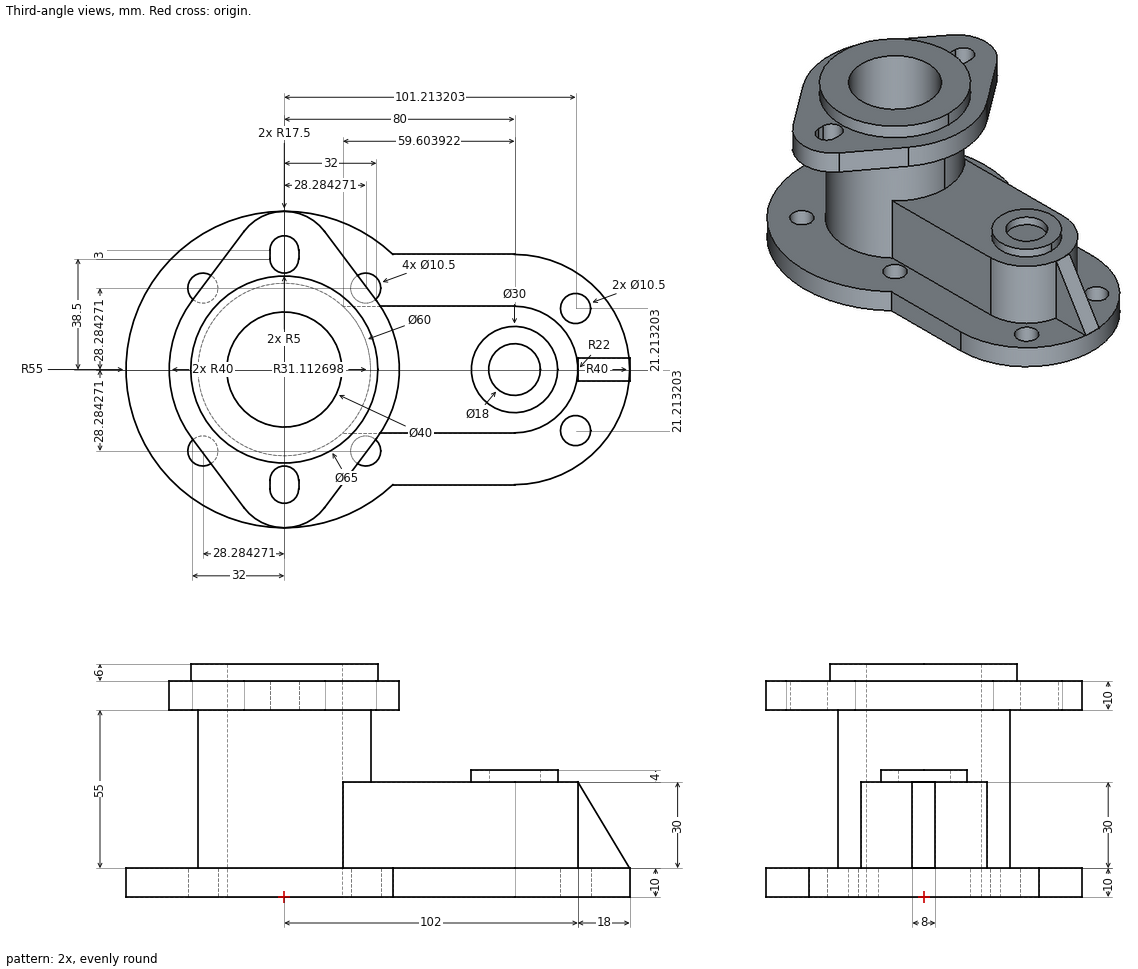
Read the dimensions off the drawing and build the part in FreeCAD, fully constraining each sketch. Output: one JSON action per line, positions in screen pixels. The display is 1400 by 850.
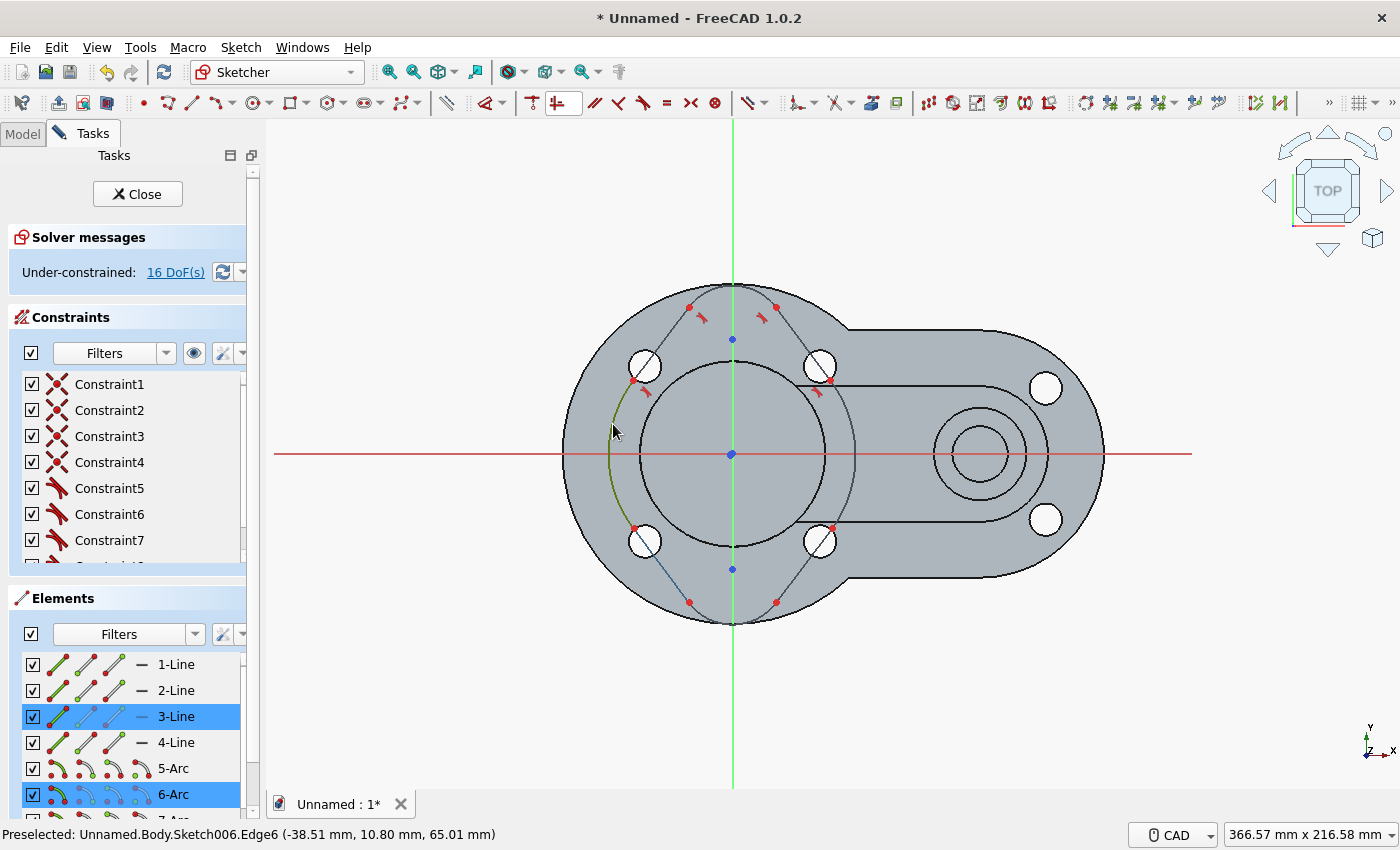
{"action": "left_click", "coordinate": [644, 104]}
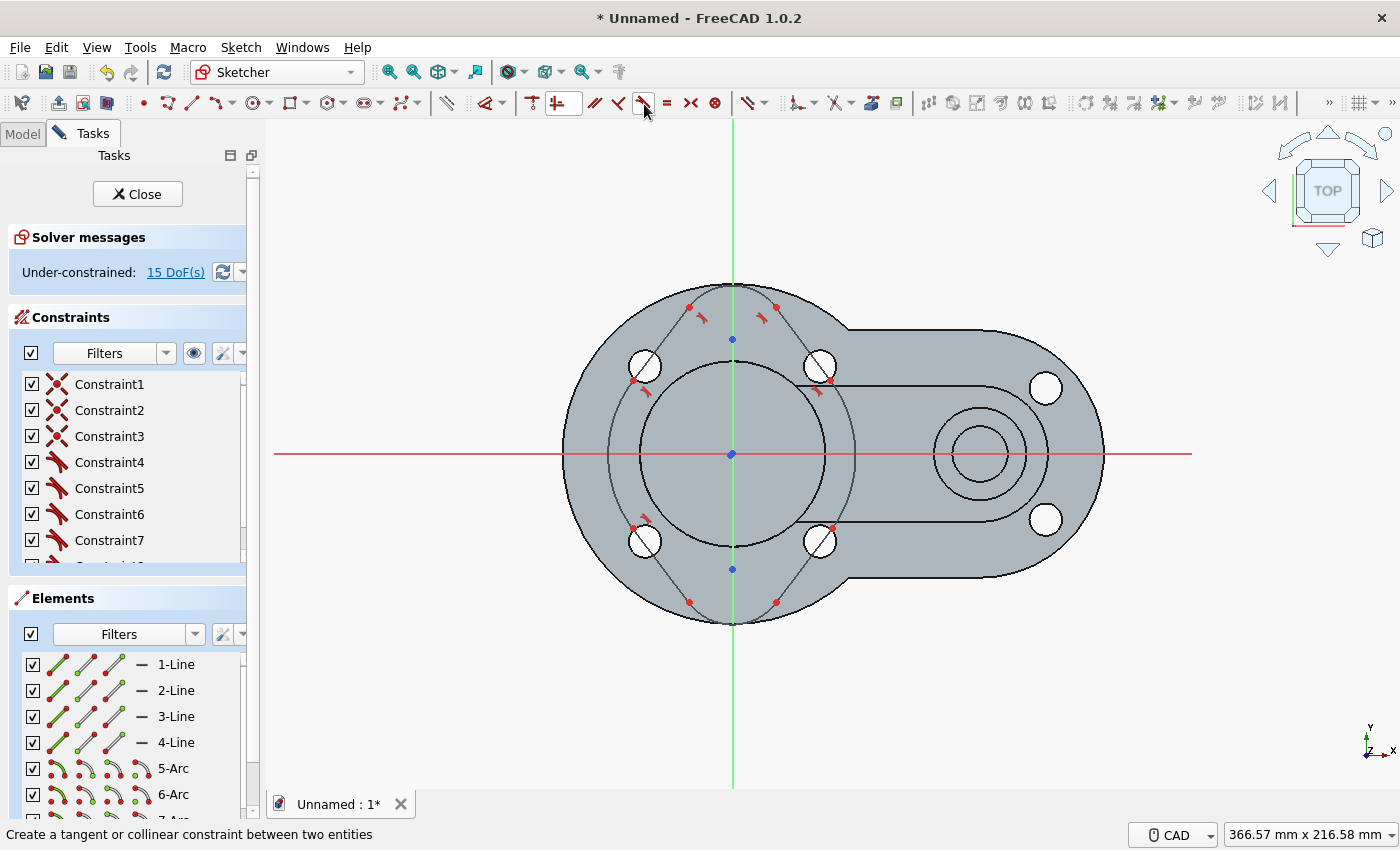
{"action": "left_click", "coordinate": [650, 551]}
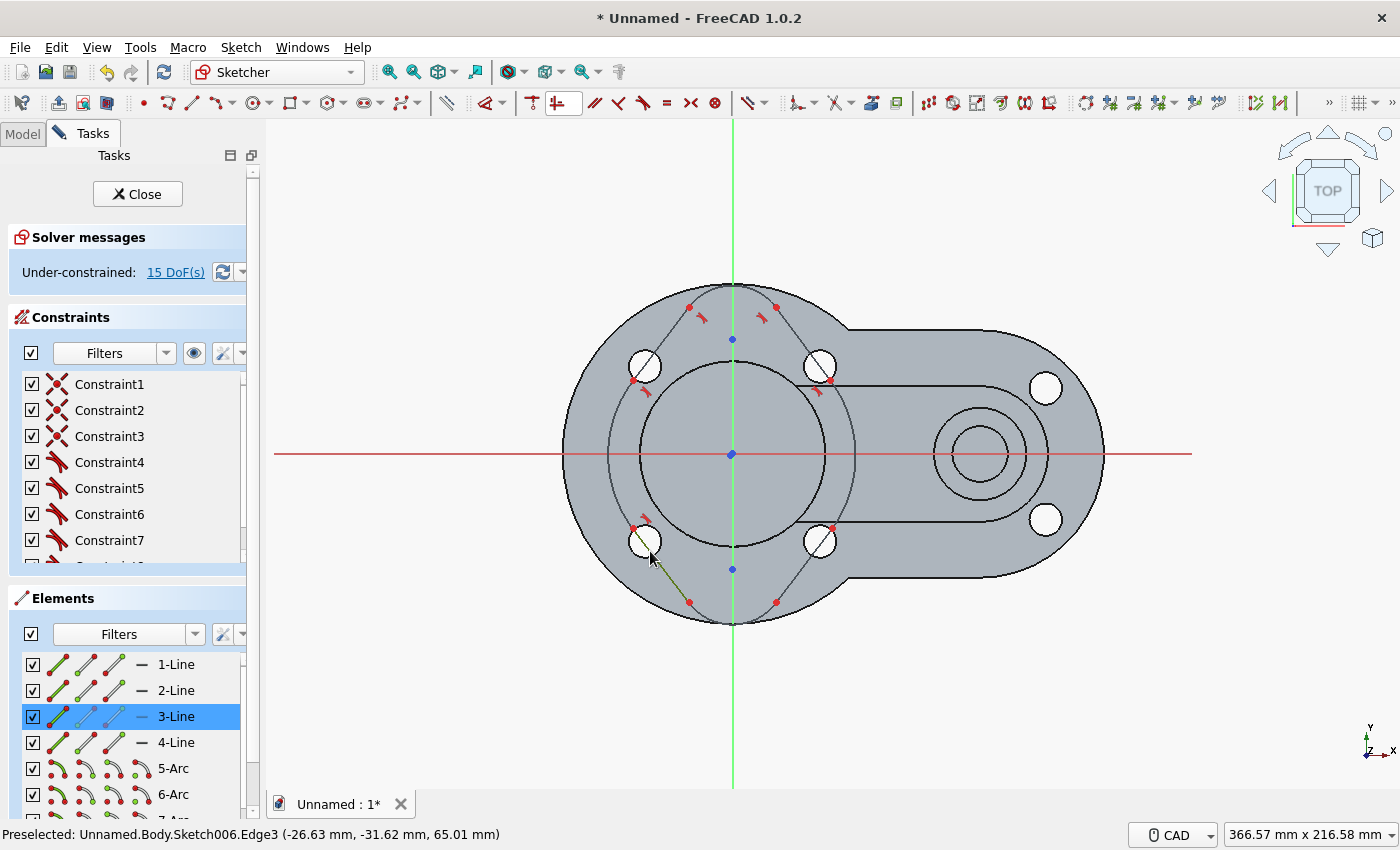
{"action": "left_click", "coordinate": [713, 621]}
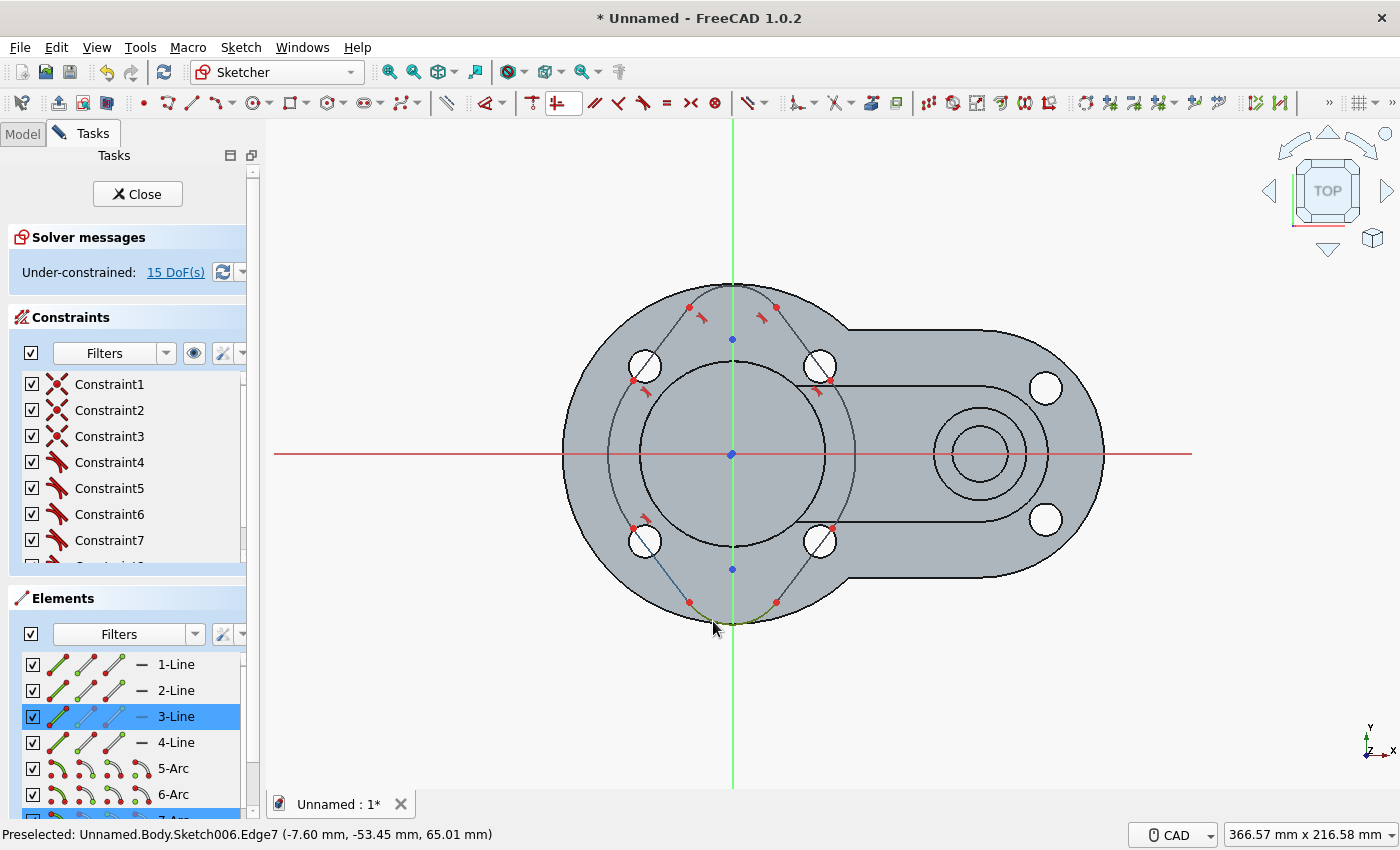
{"action": "key", "text": "t"}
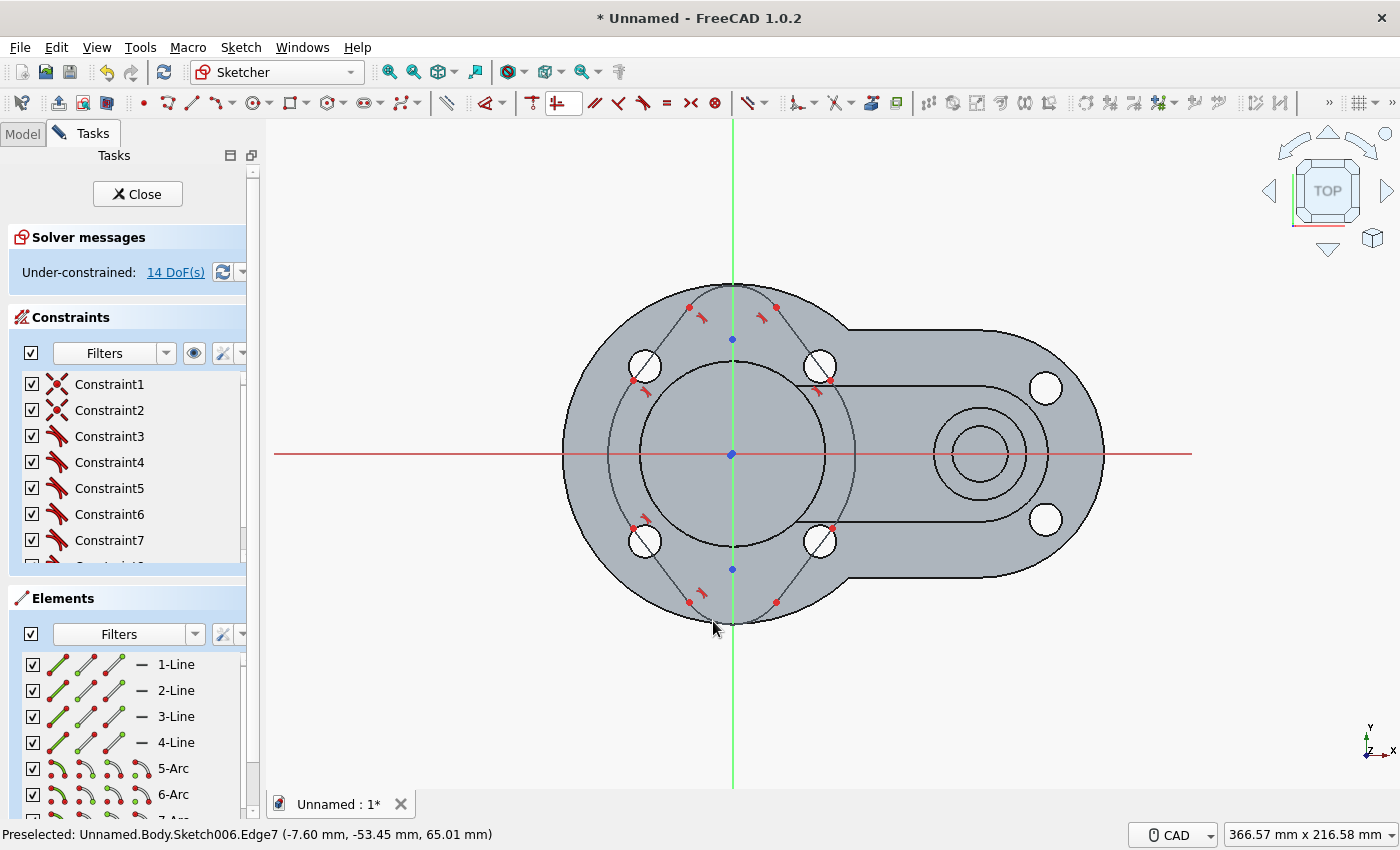
{"action": "left_click", "coordinate": [793, 581]}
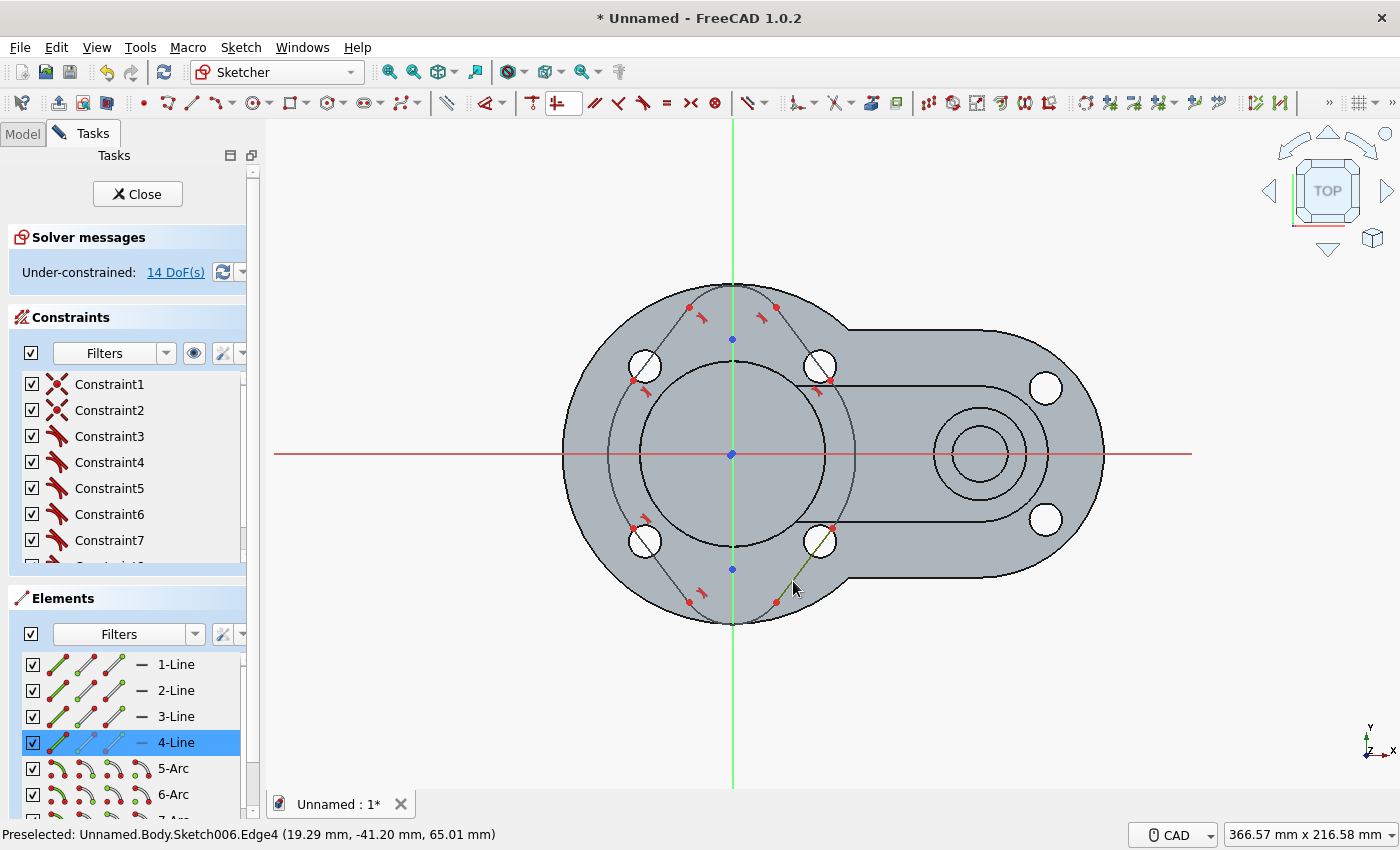
{"action": "left_click", "coordinate": [713, 621]}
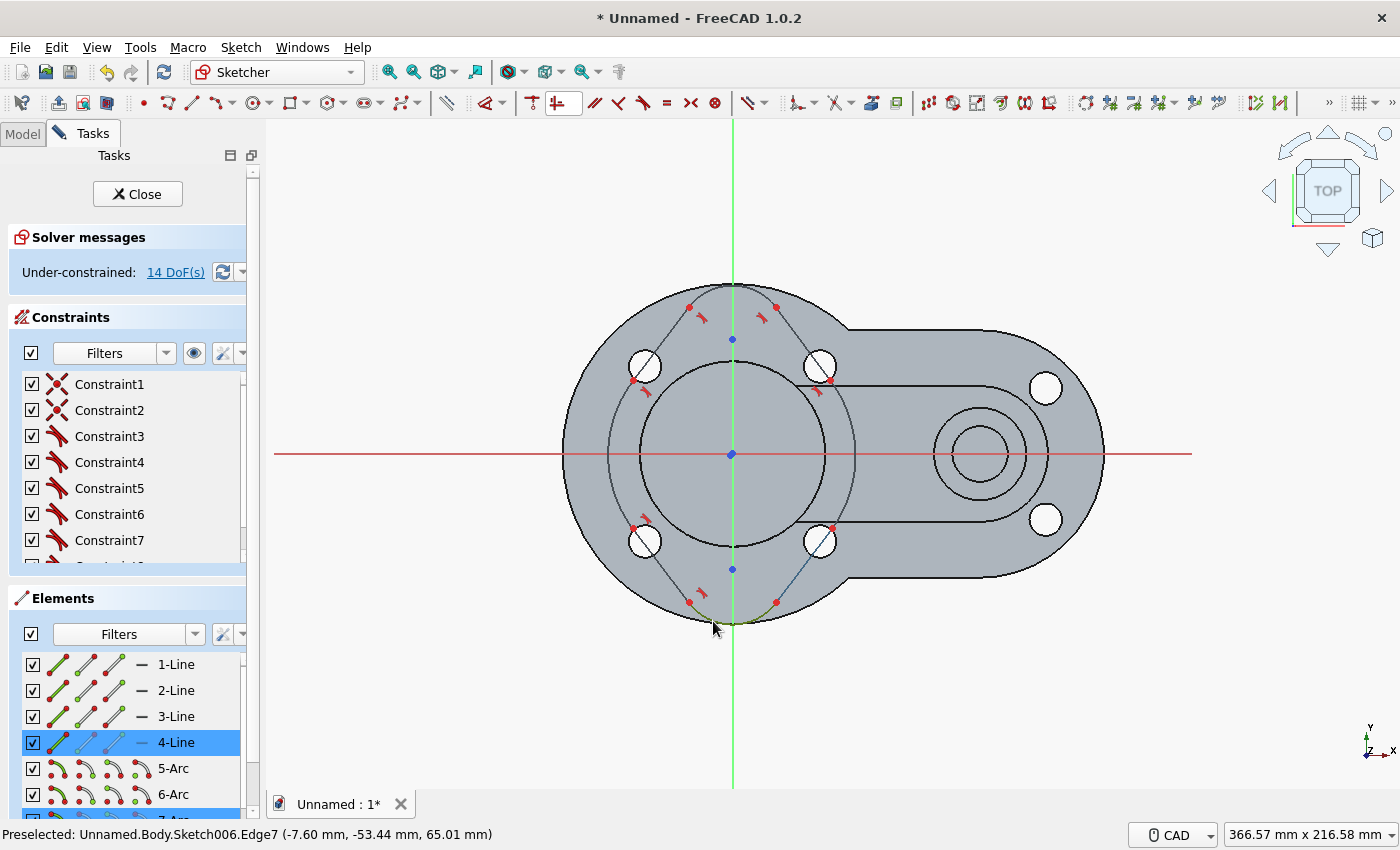
{"action": "key", "text": "t"}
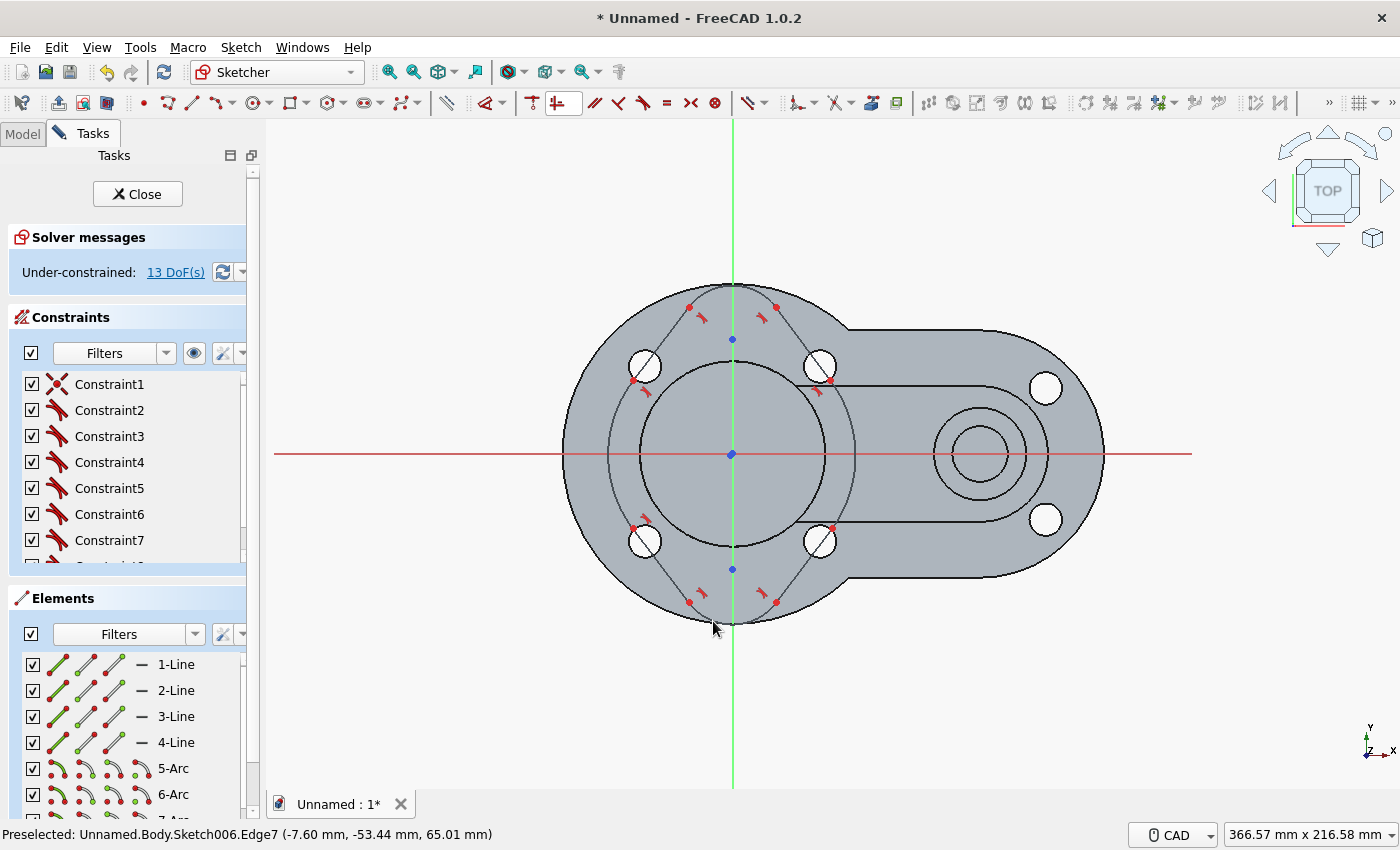
{"action": "left_click", "coordinate": [793, 581]}